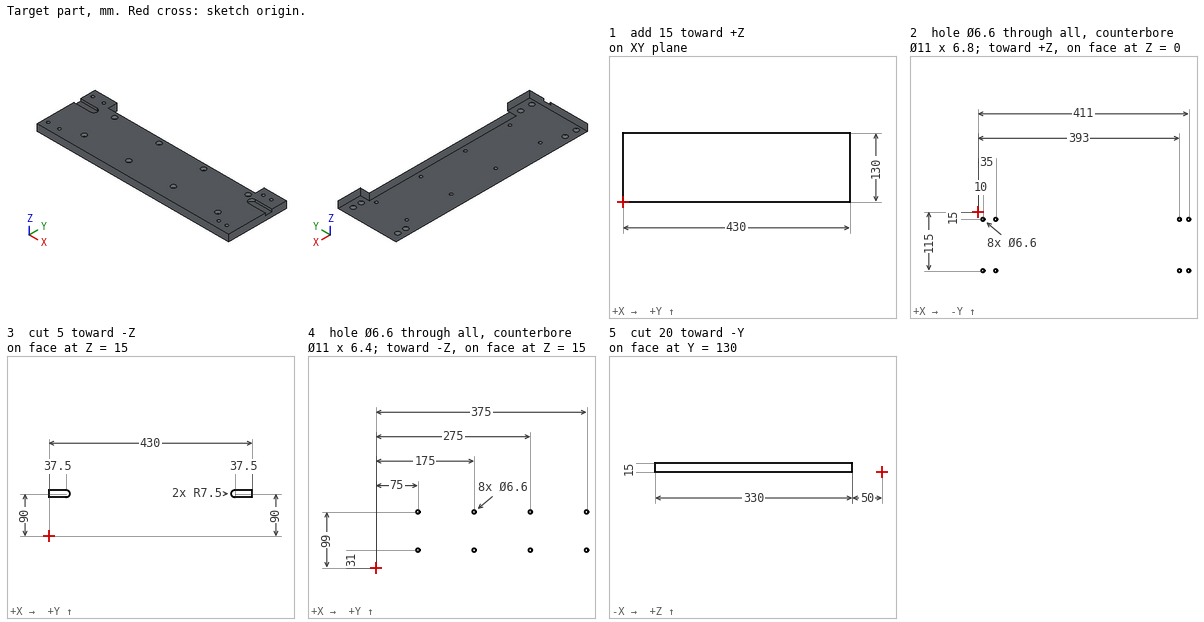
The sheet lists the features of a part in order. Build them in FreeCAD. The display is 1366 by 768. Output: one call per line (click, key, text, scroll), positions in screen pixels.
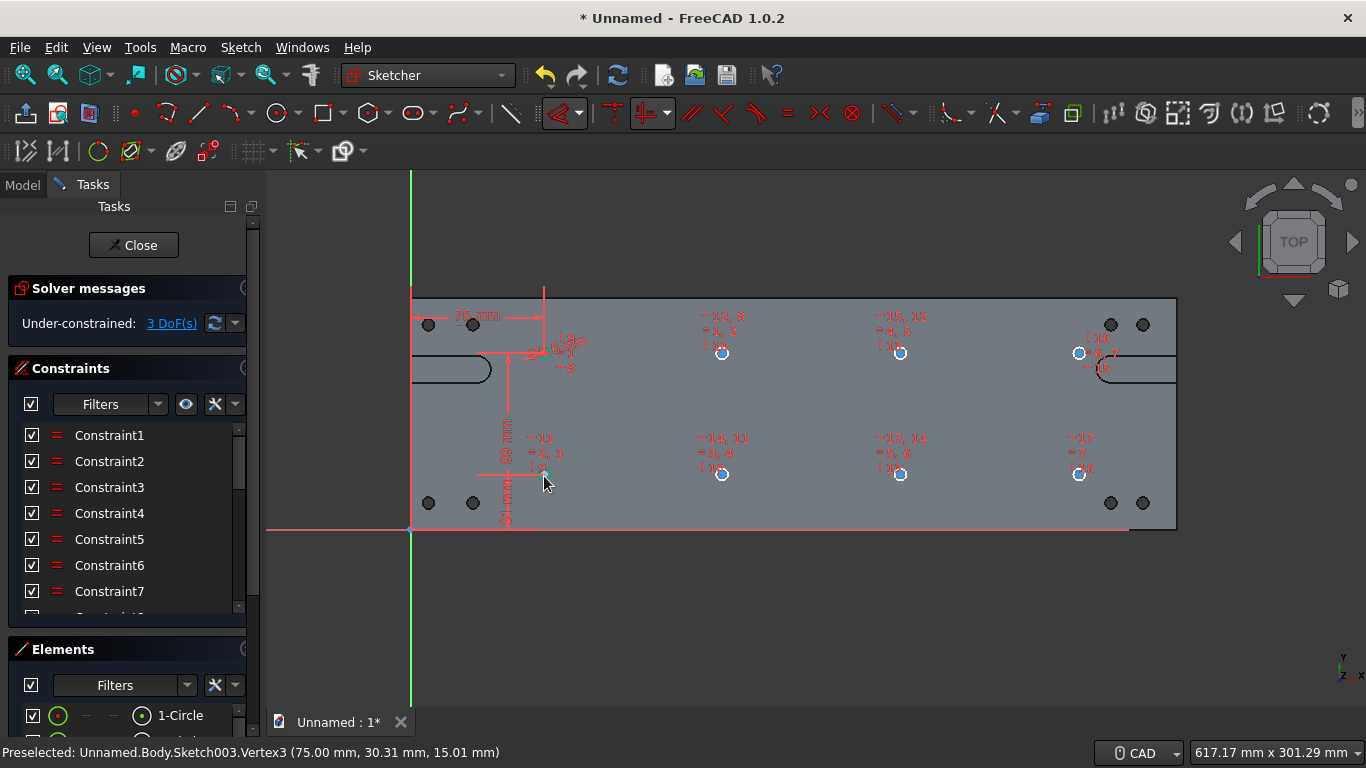
click(722, 353)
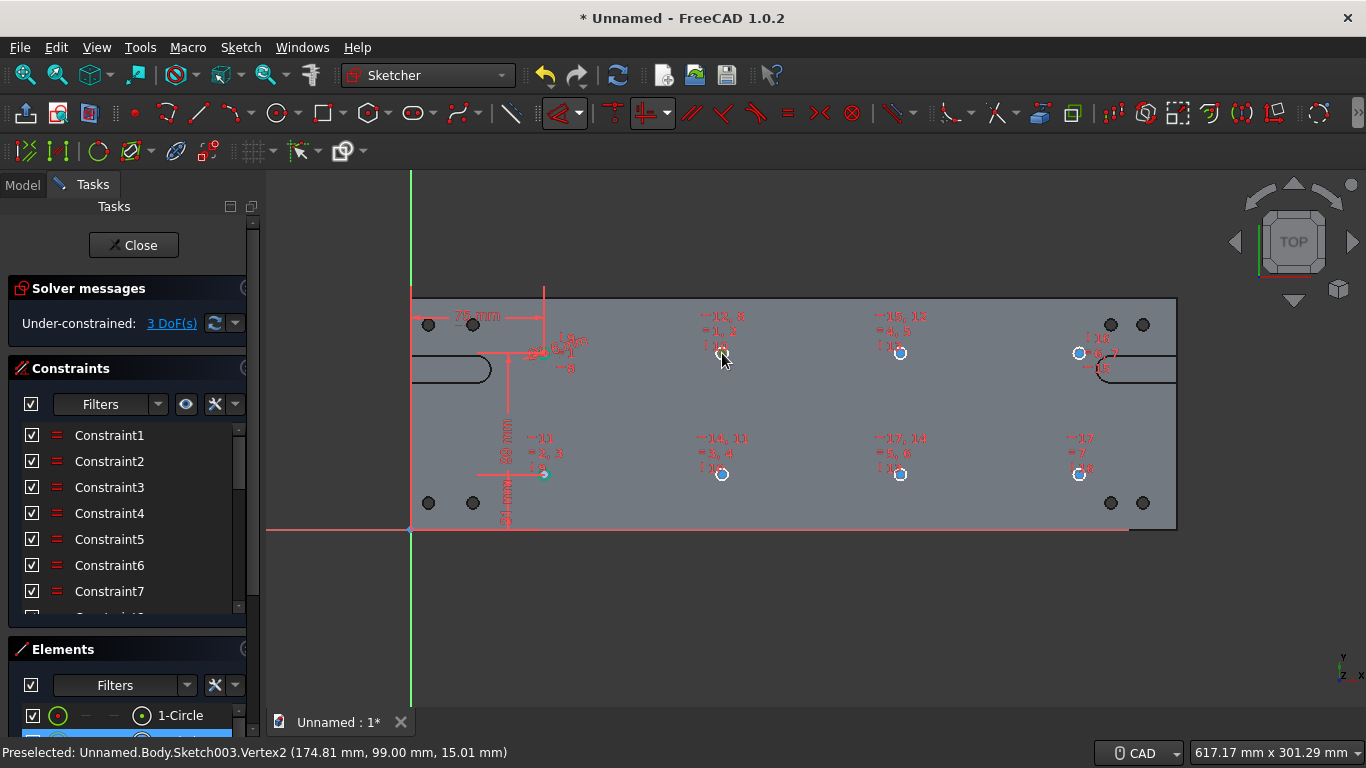
click(582, 114)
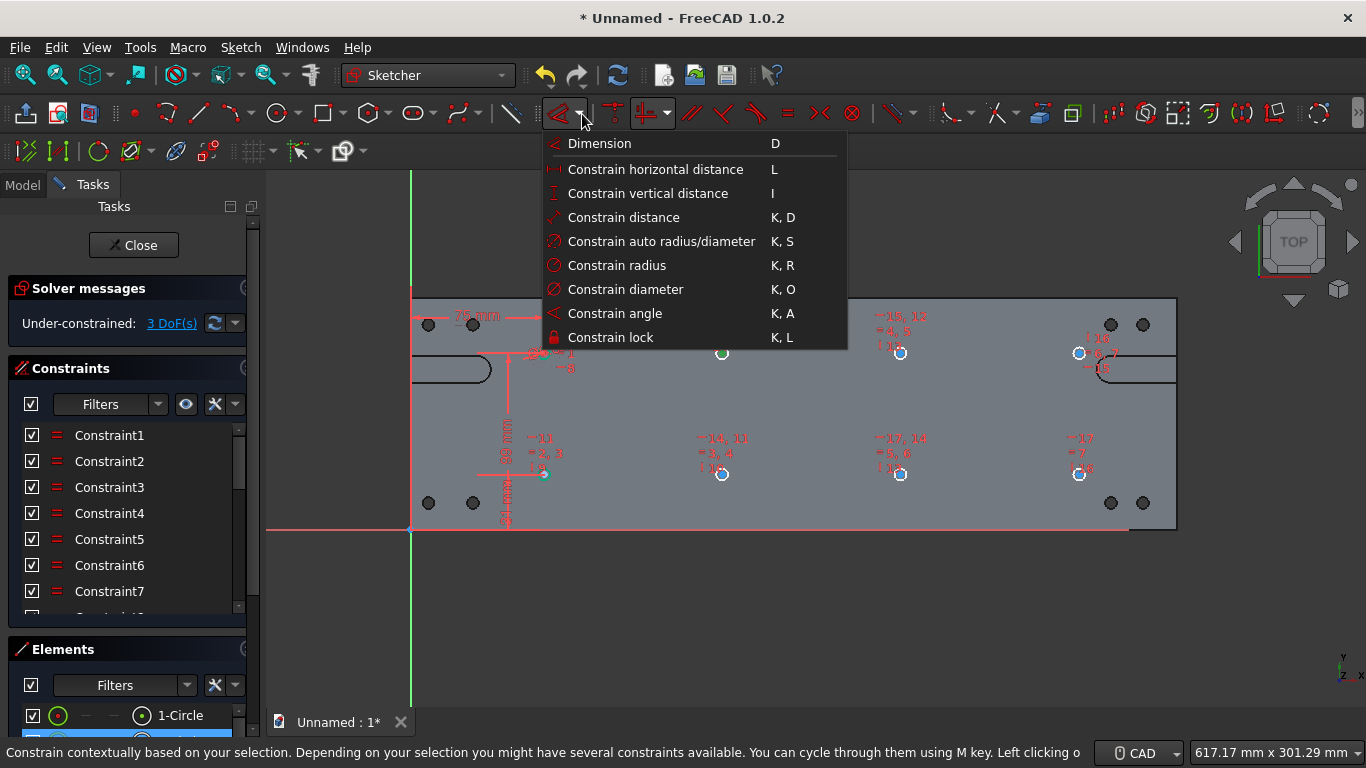
click(695, 169)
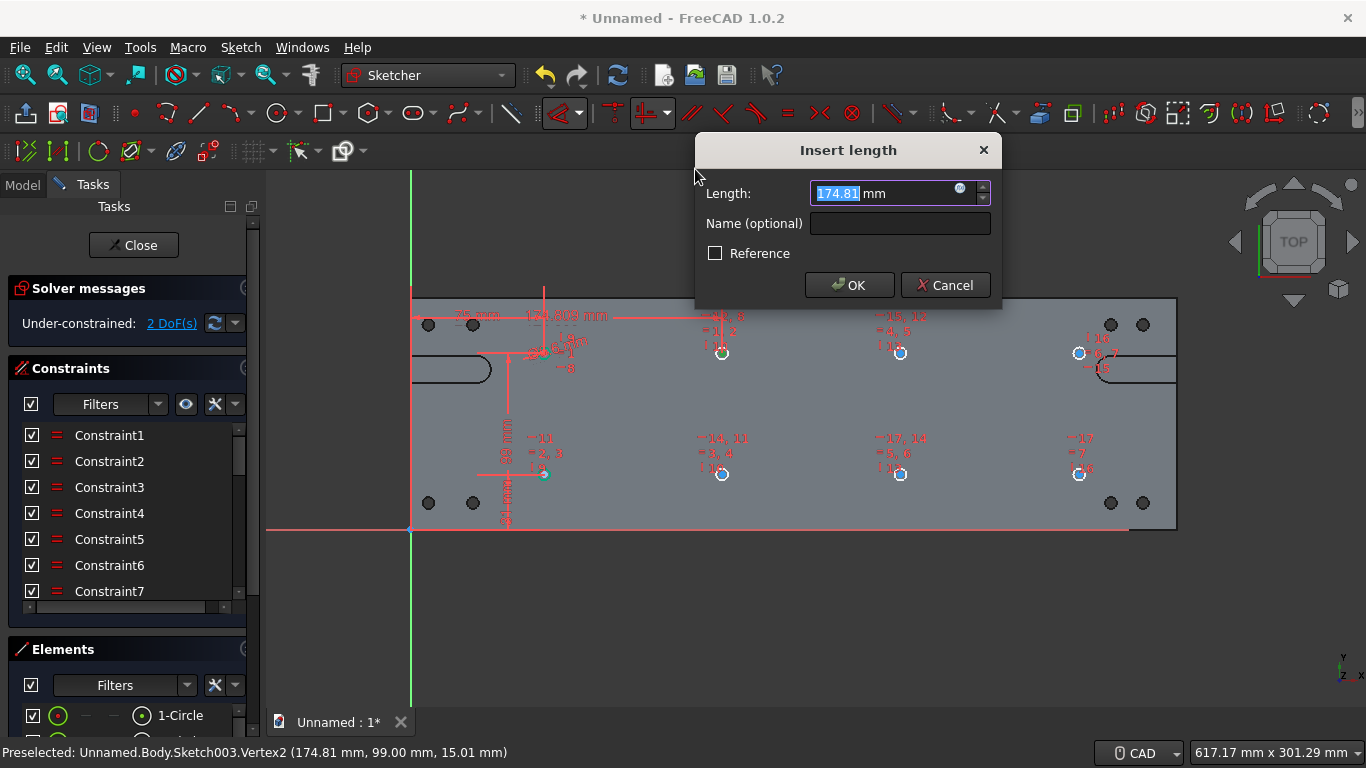
text(175)
key(Return)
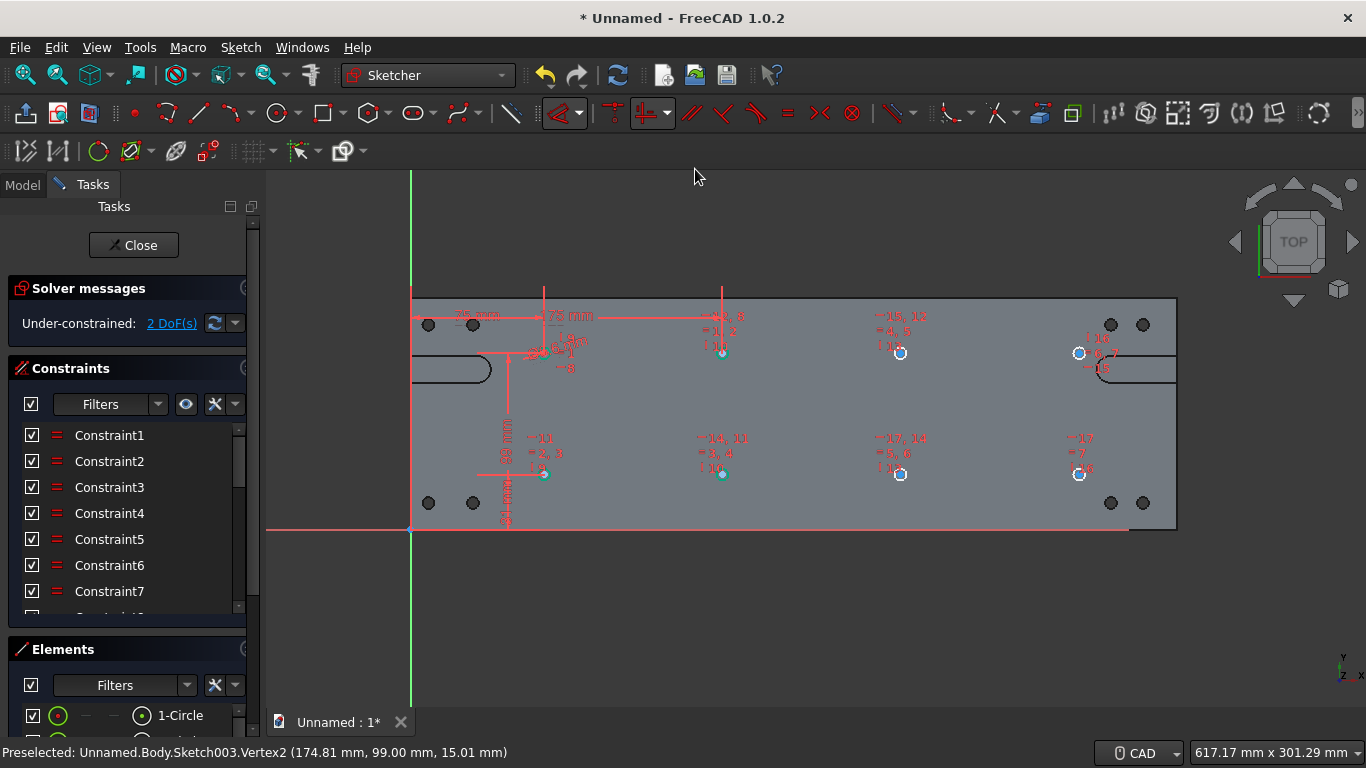
click(900, 353)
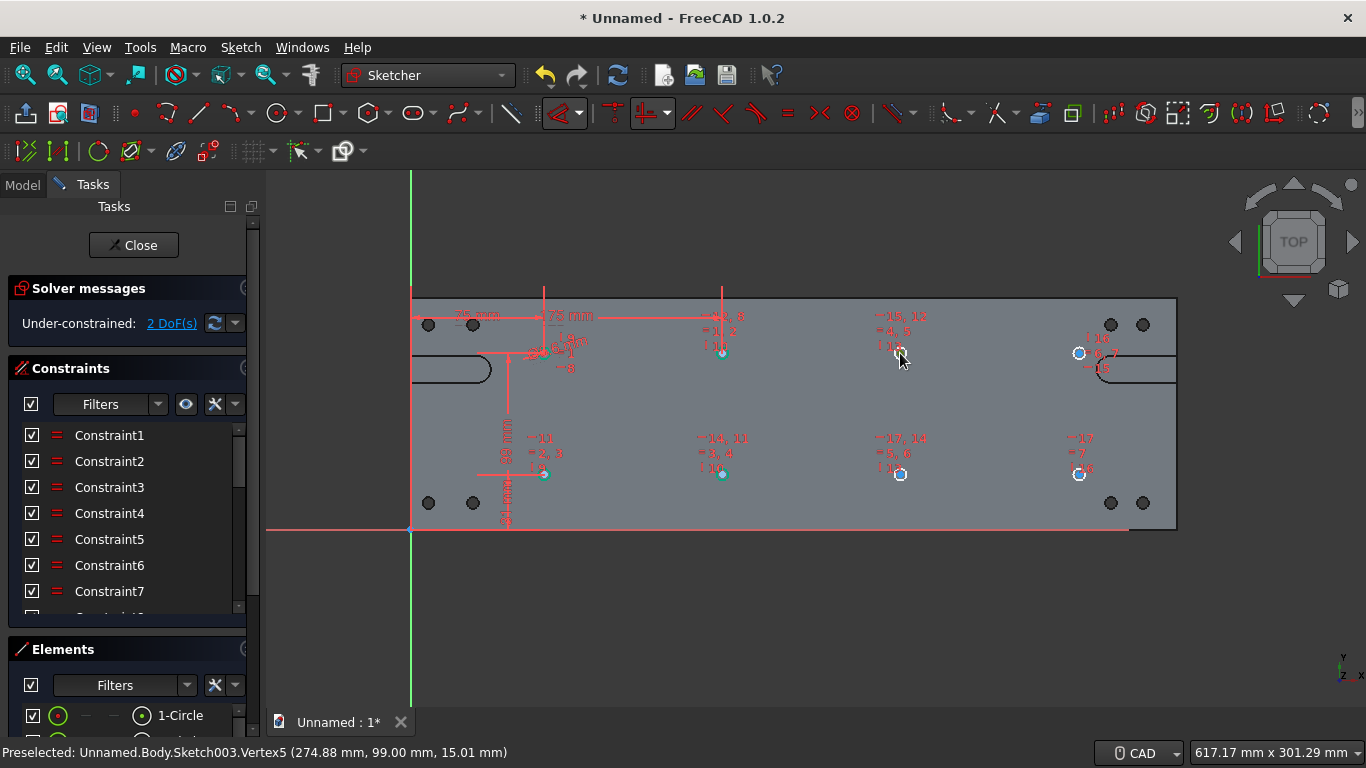
key(l)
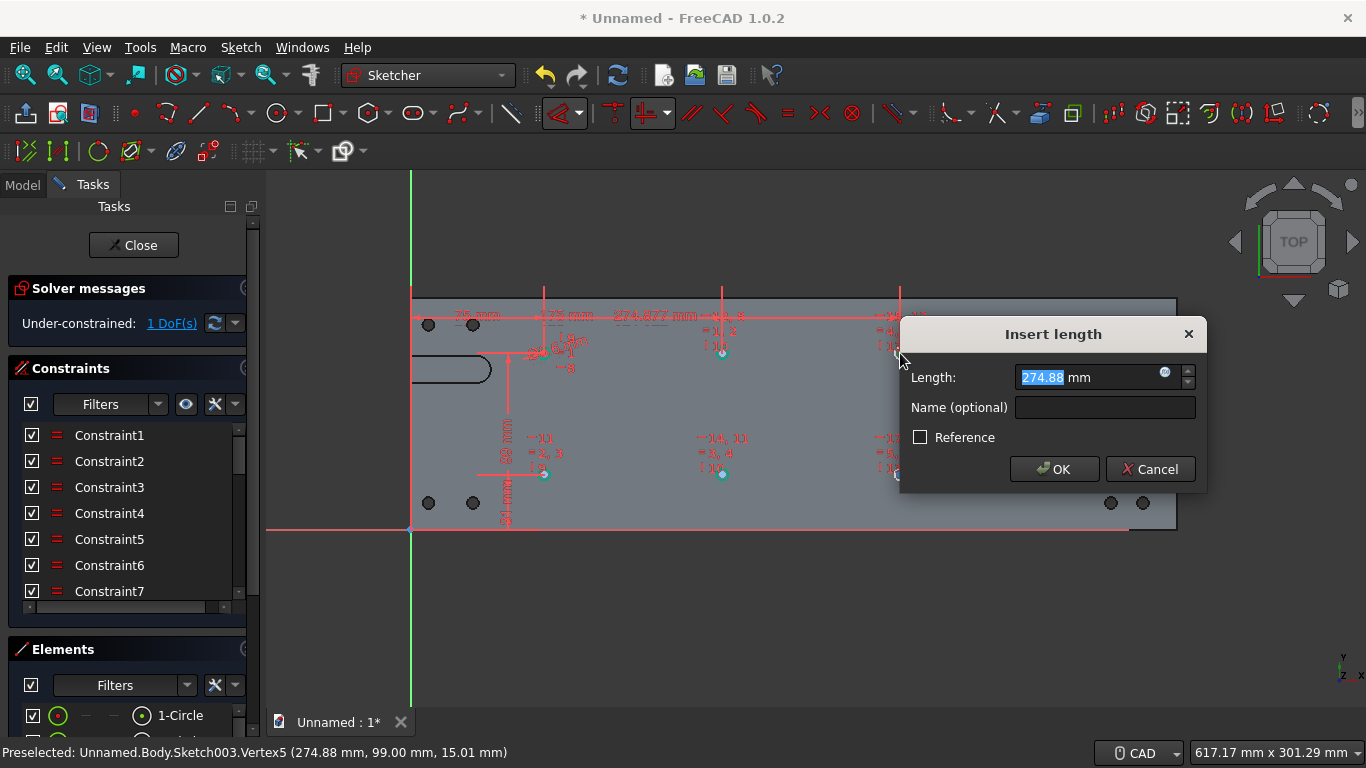
text(275)
key(Return)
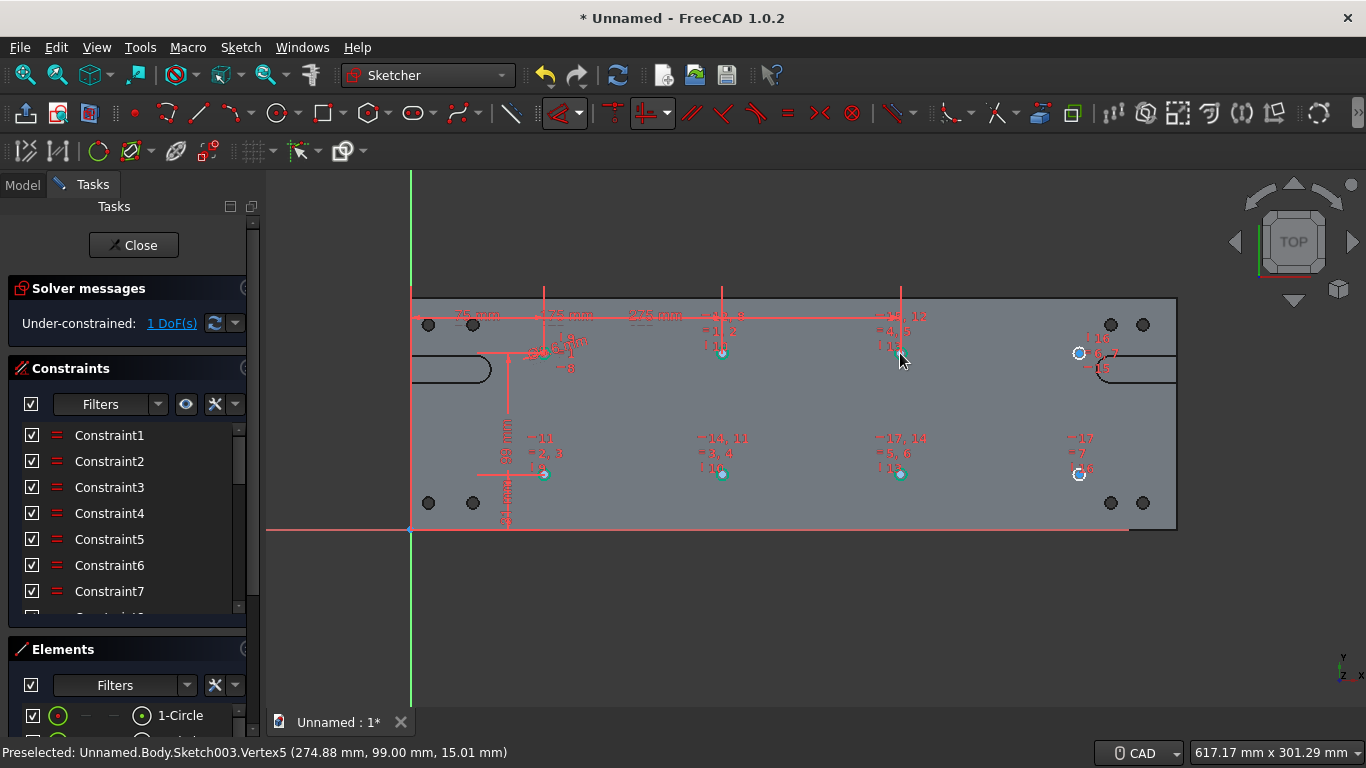
click(1079, 353)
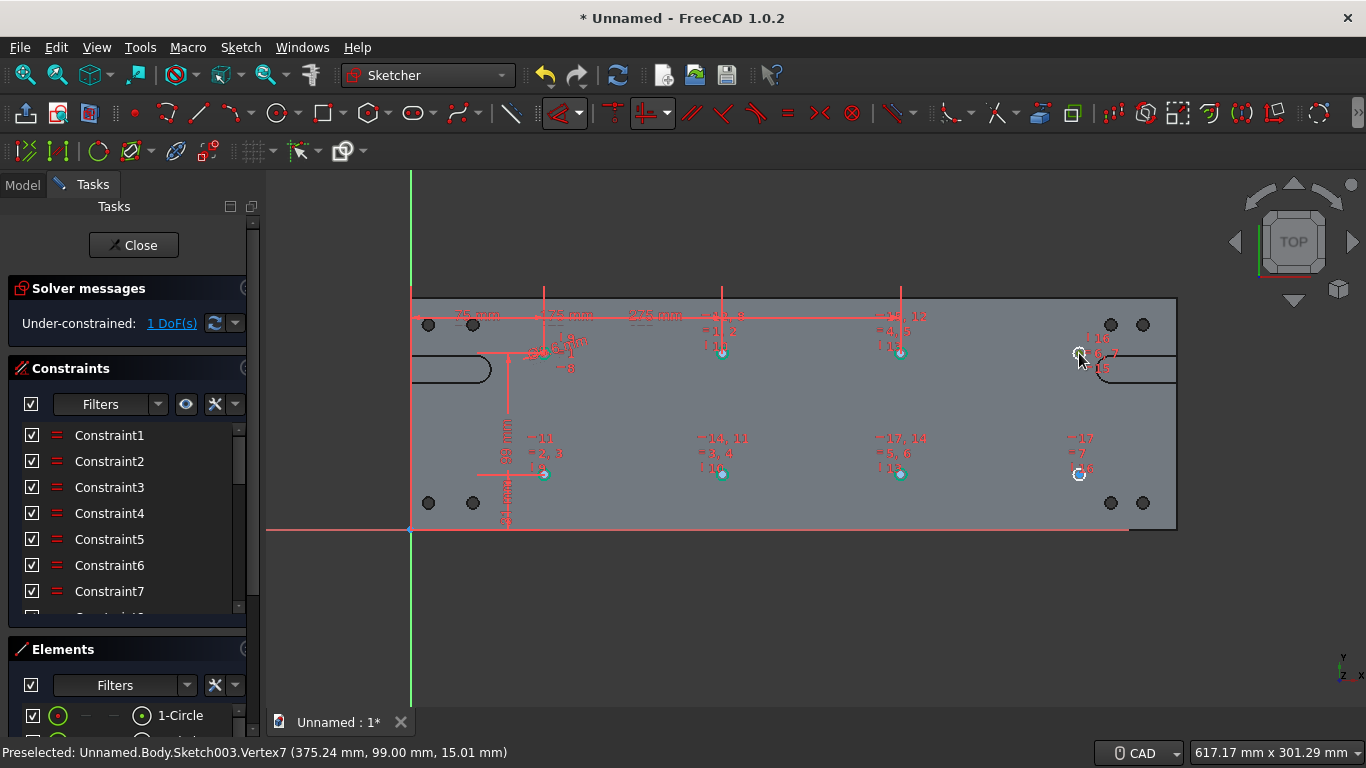
click(582, 114)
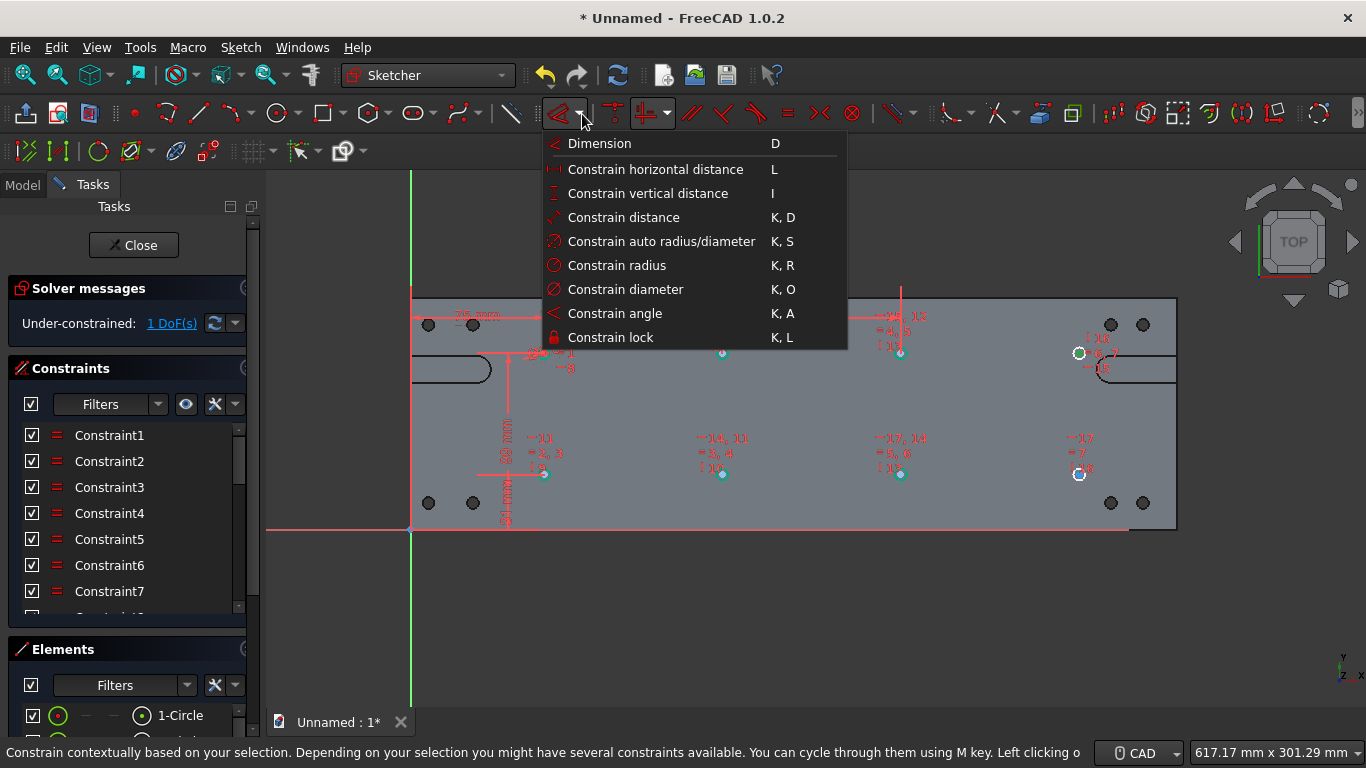
click(695, 169)